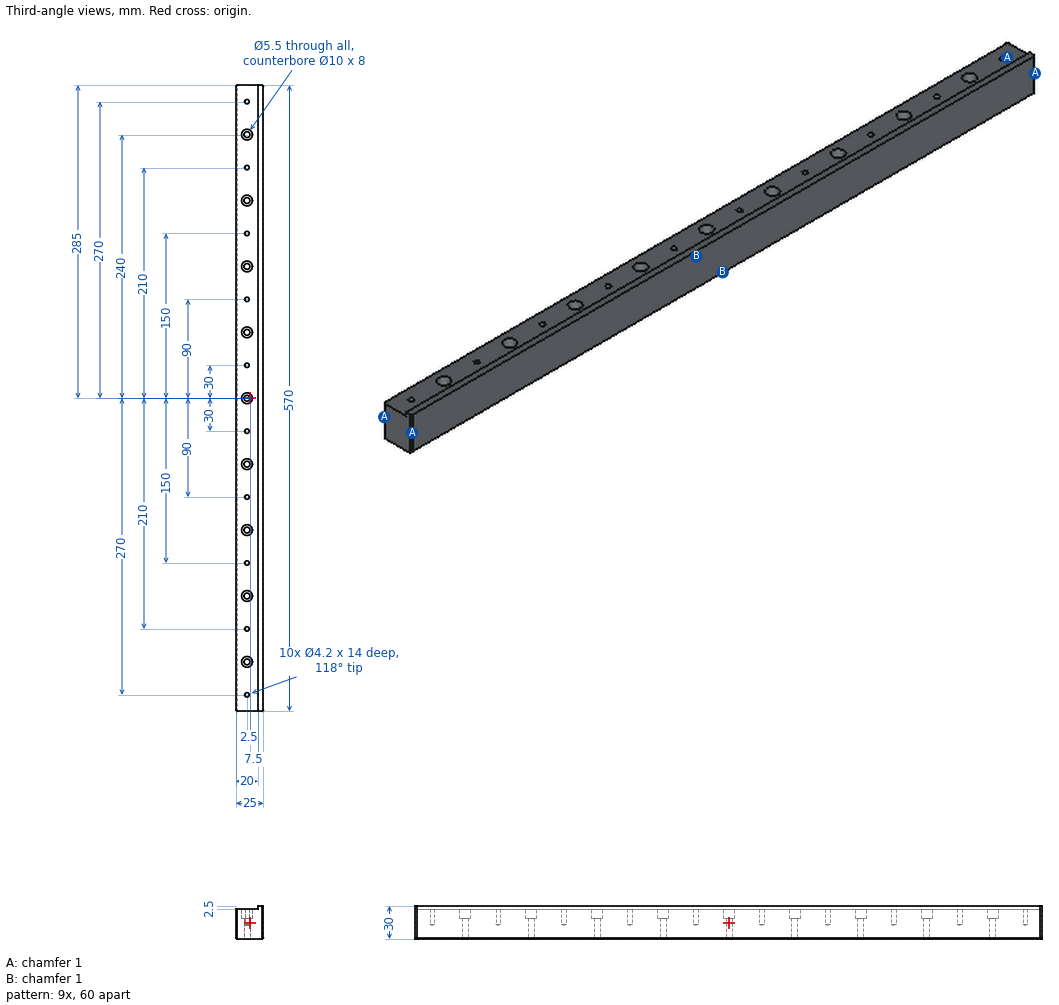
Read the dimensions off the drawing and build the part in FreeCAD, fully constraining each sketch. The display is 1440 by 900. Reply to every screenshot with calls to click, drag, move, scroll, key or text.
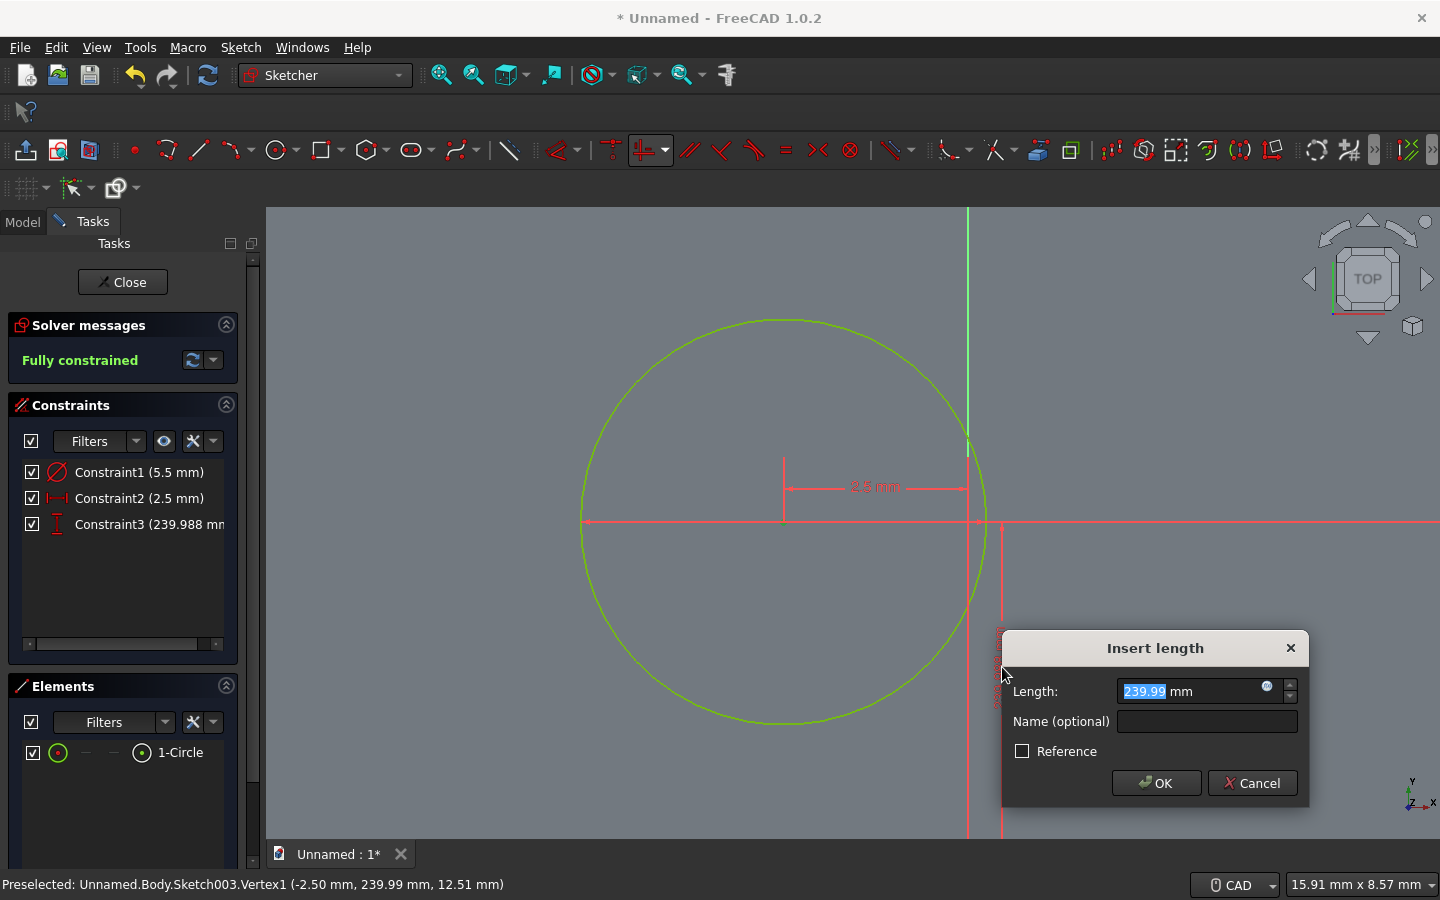
text(240)
key(Return)
key(Escape)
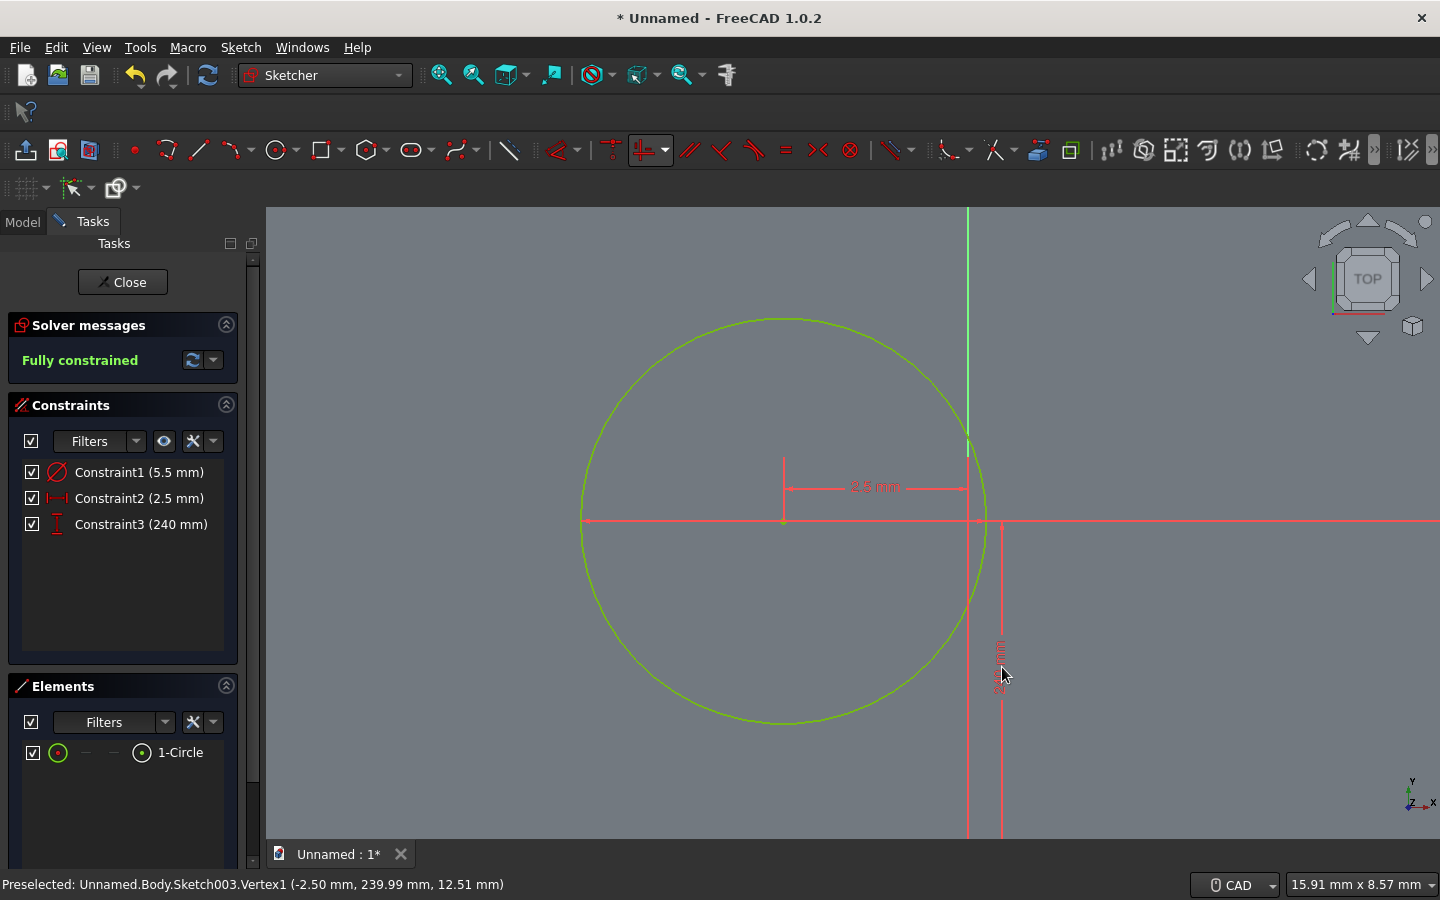
click(123, 282)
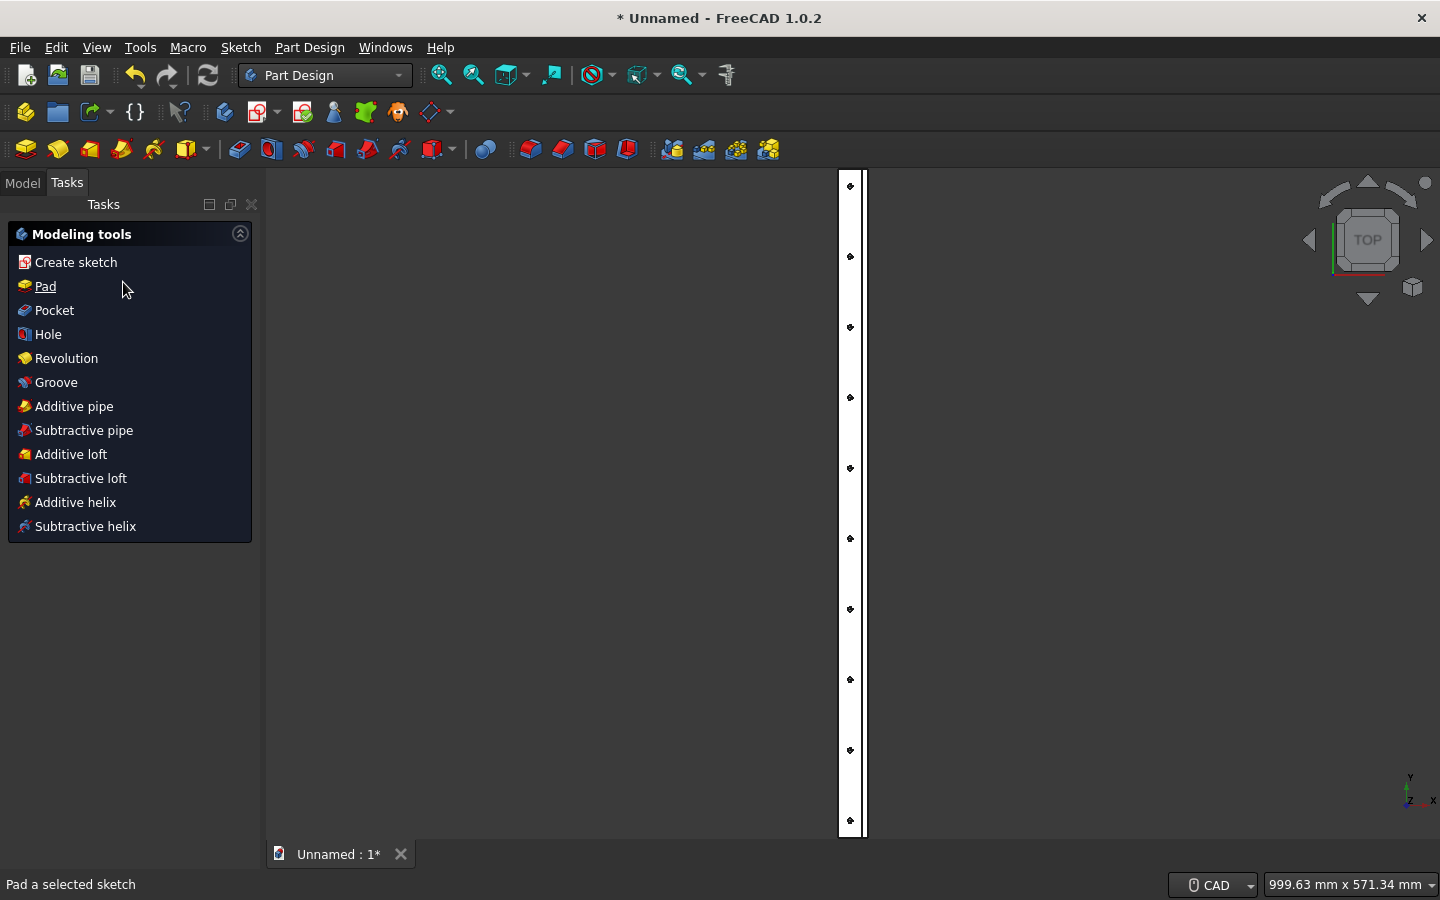
click(272, 150)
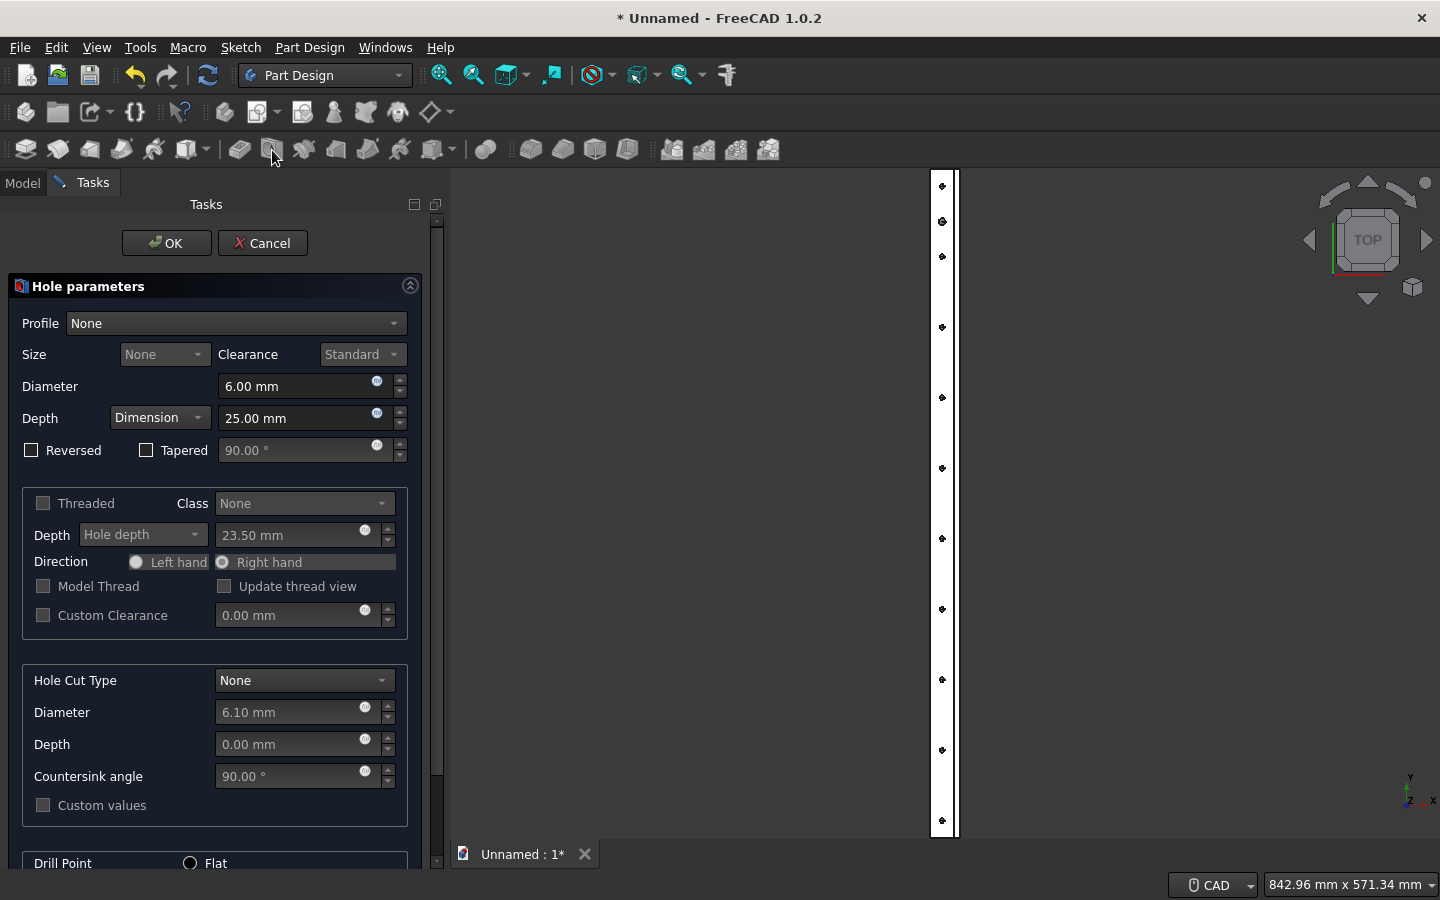
triple_click(305, 386)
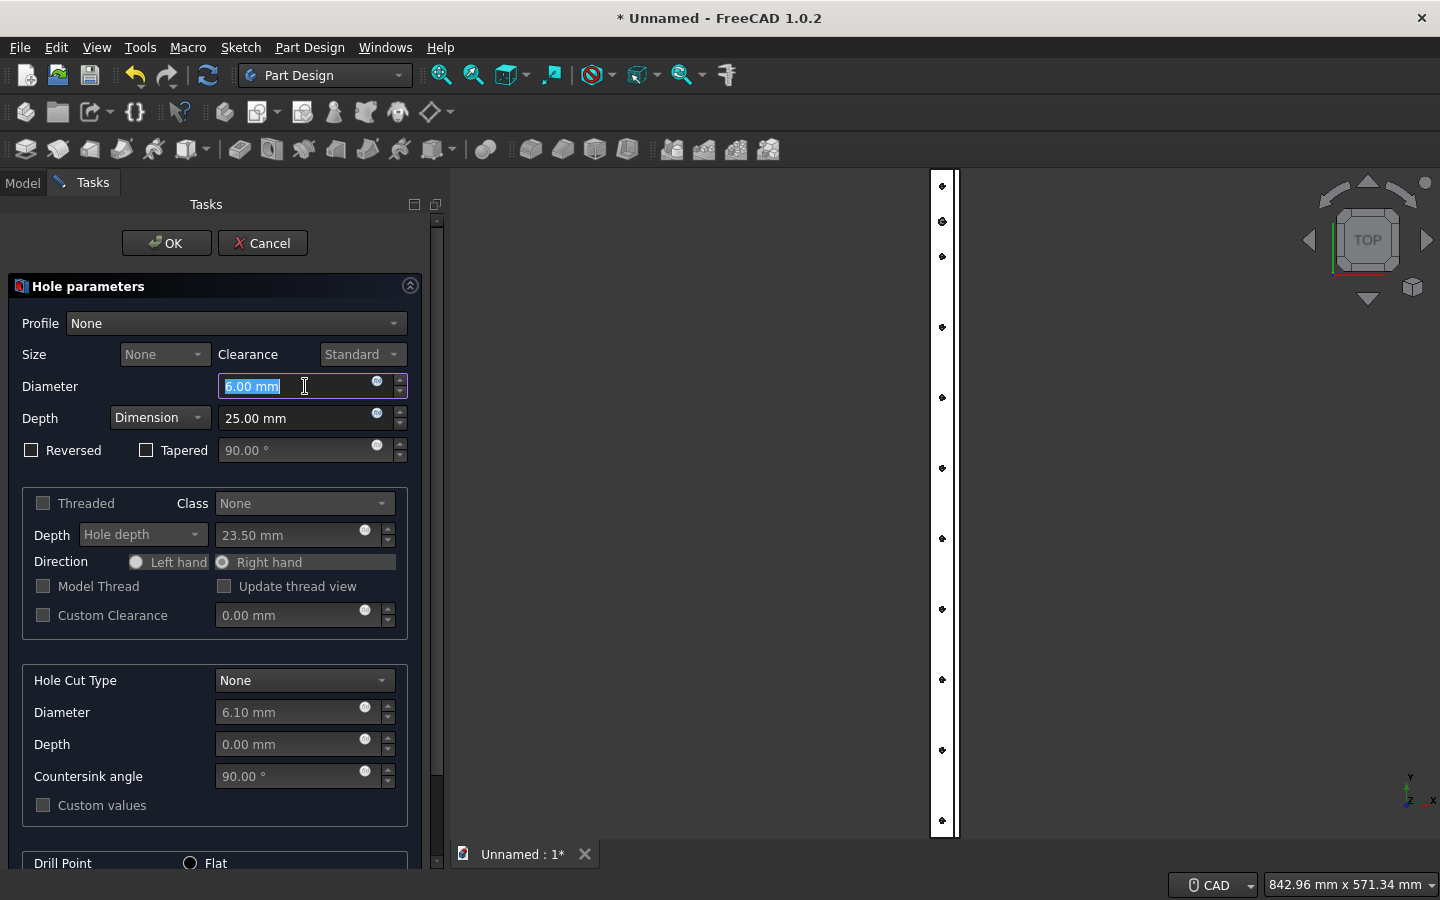
text(5.5)
key(Tab)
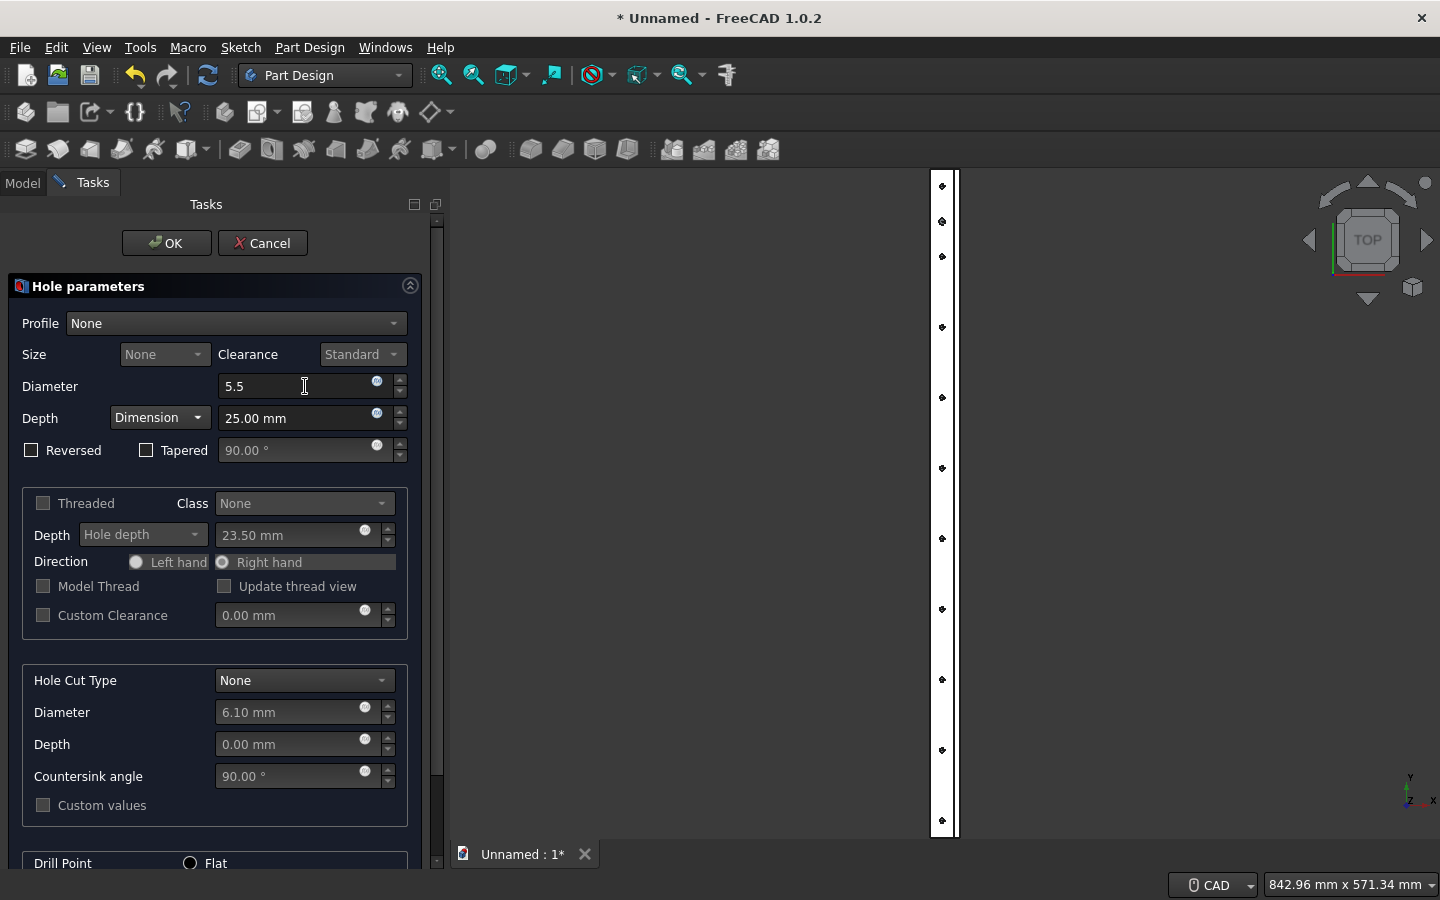
click(161, 418)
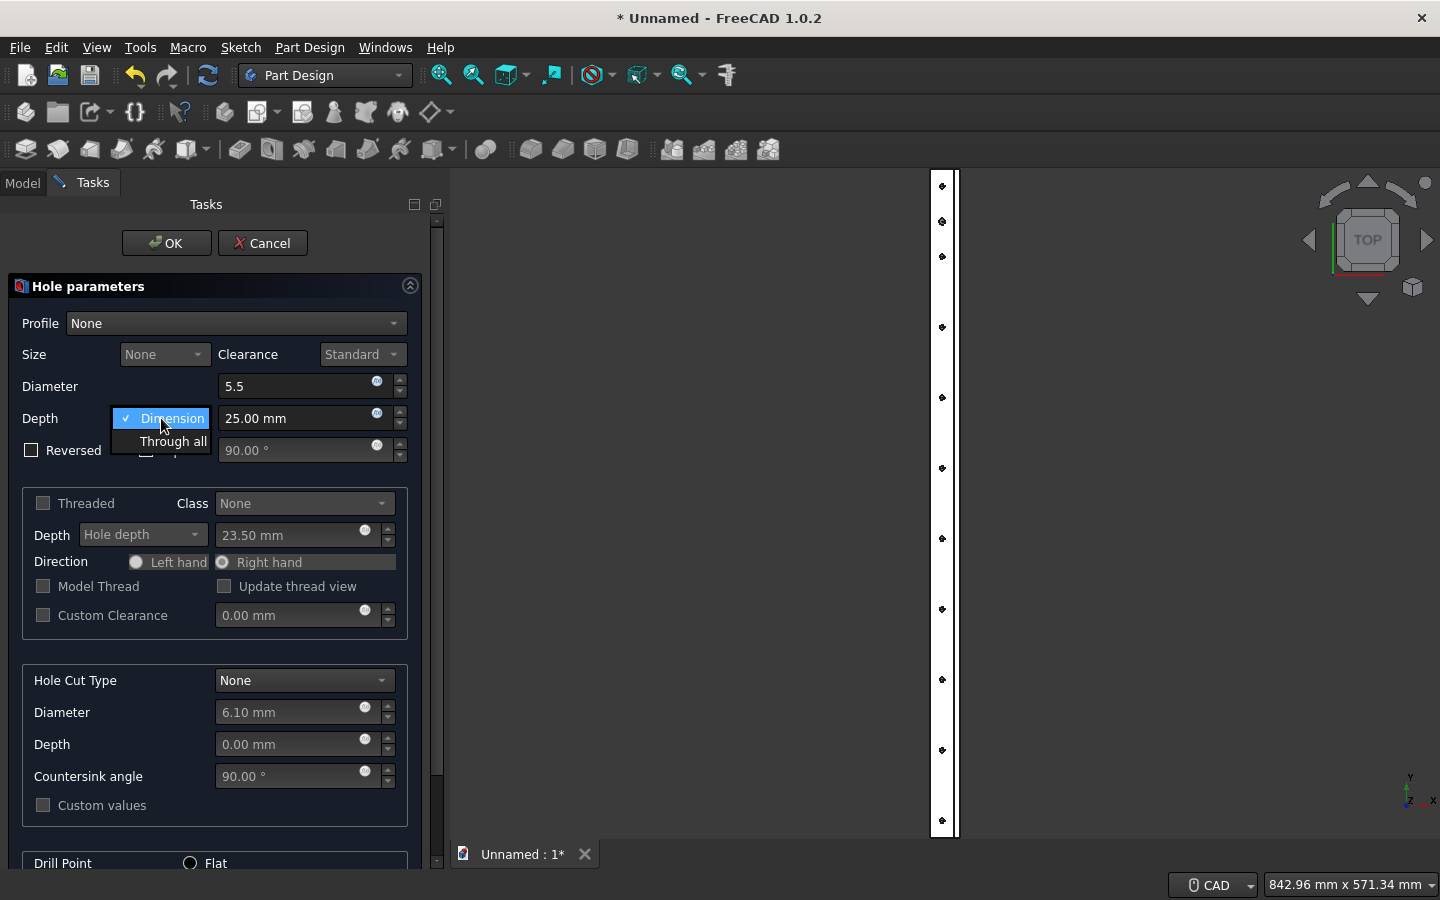
click(160, 442)